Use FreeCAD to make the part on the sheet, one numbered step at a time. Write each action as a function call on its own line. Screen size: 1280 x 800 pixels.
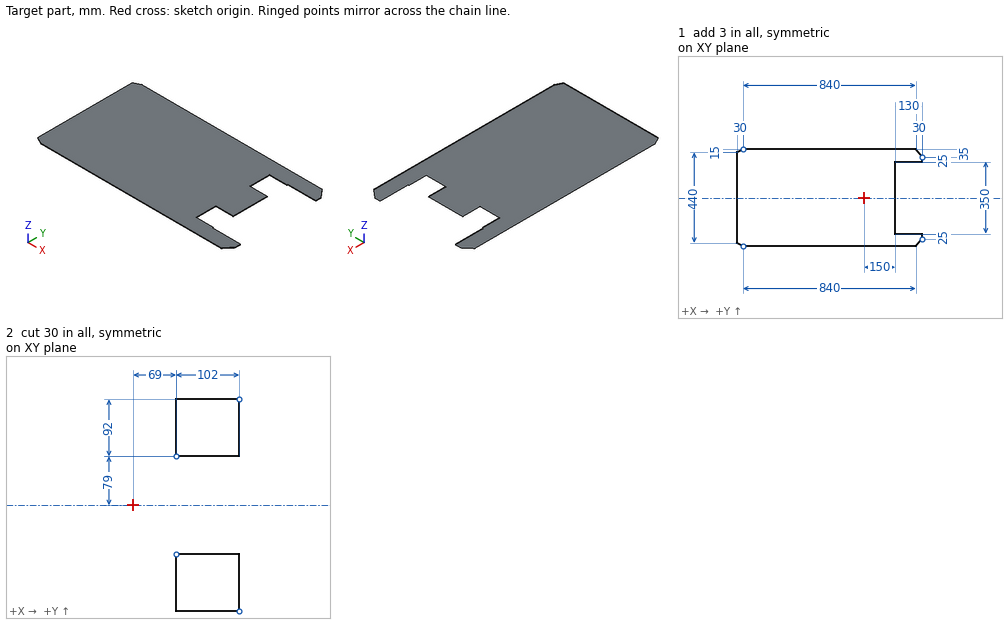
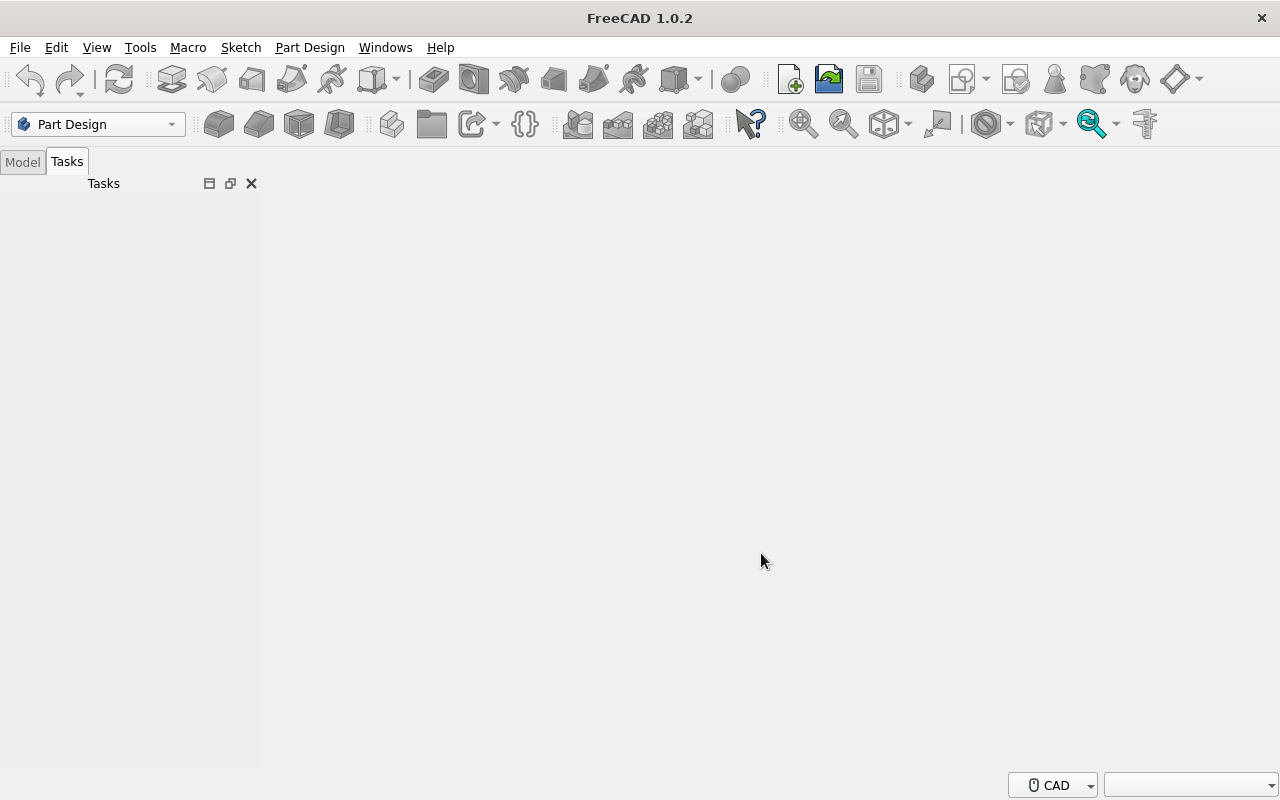
click(790, 80)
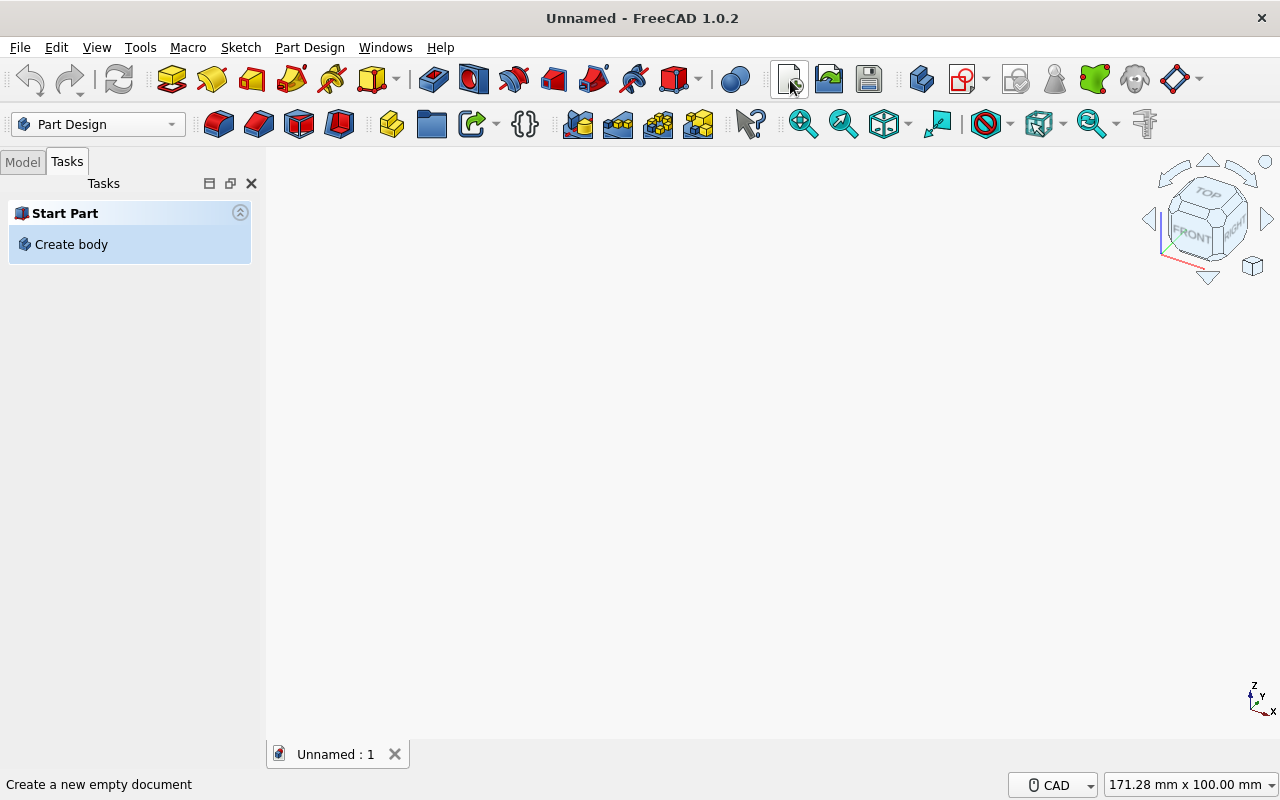
click(962, 80)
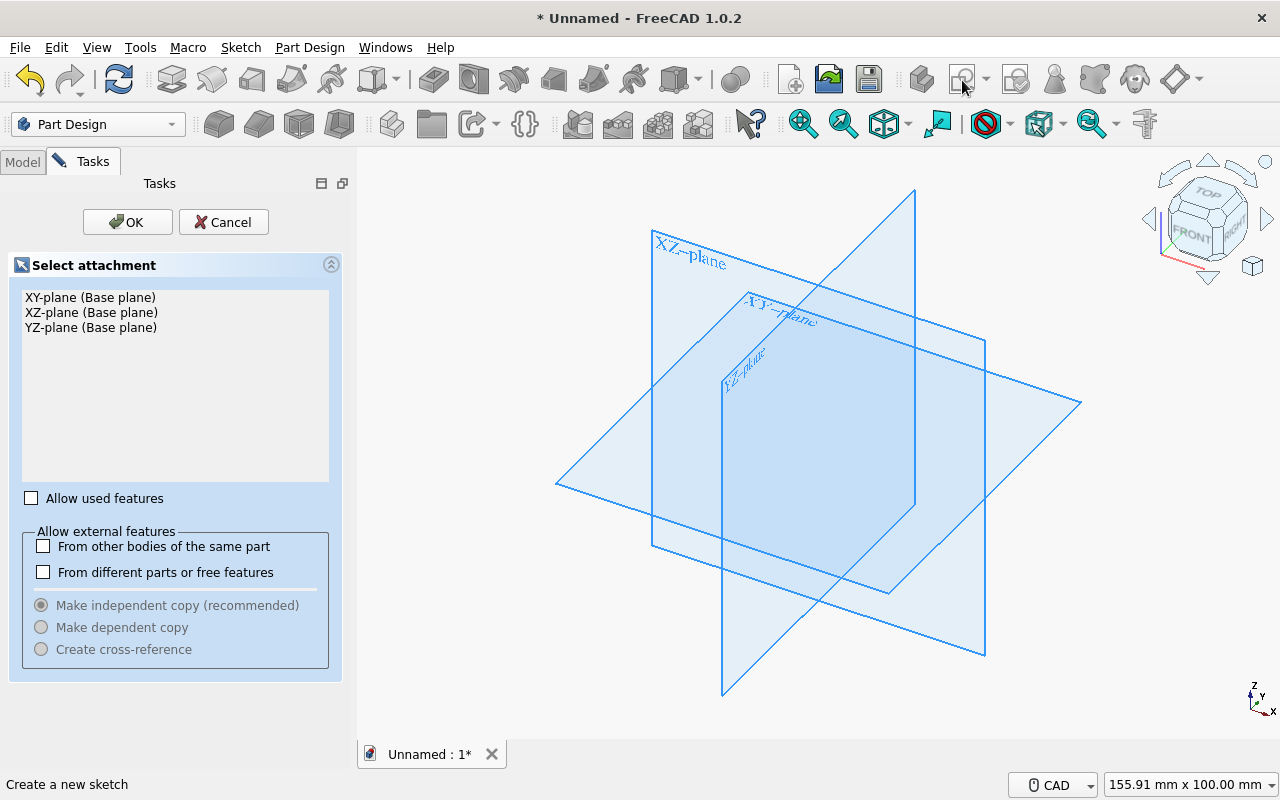
click(82, 298)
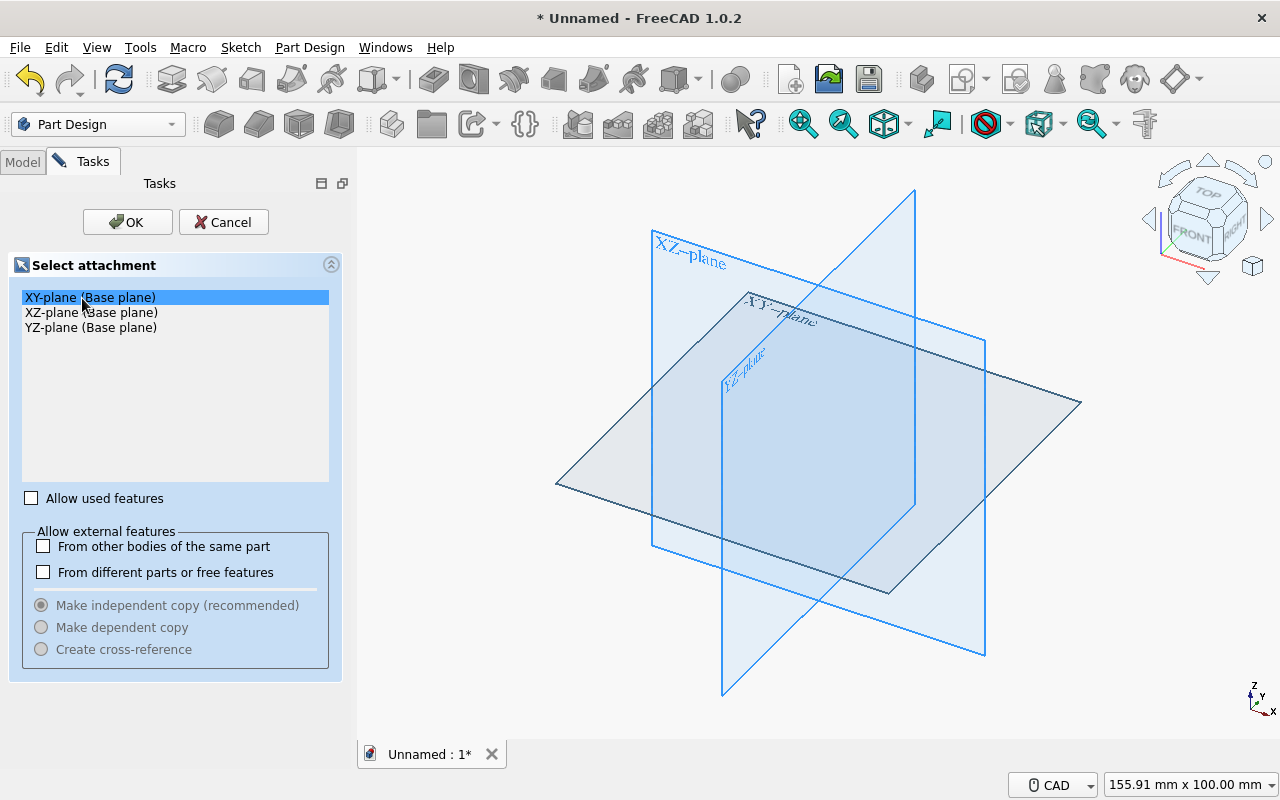
click(128, 222)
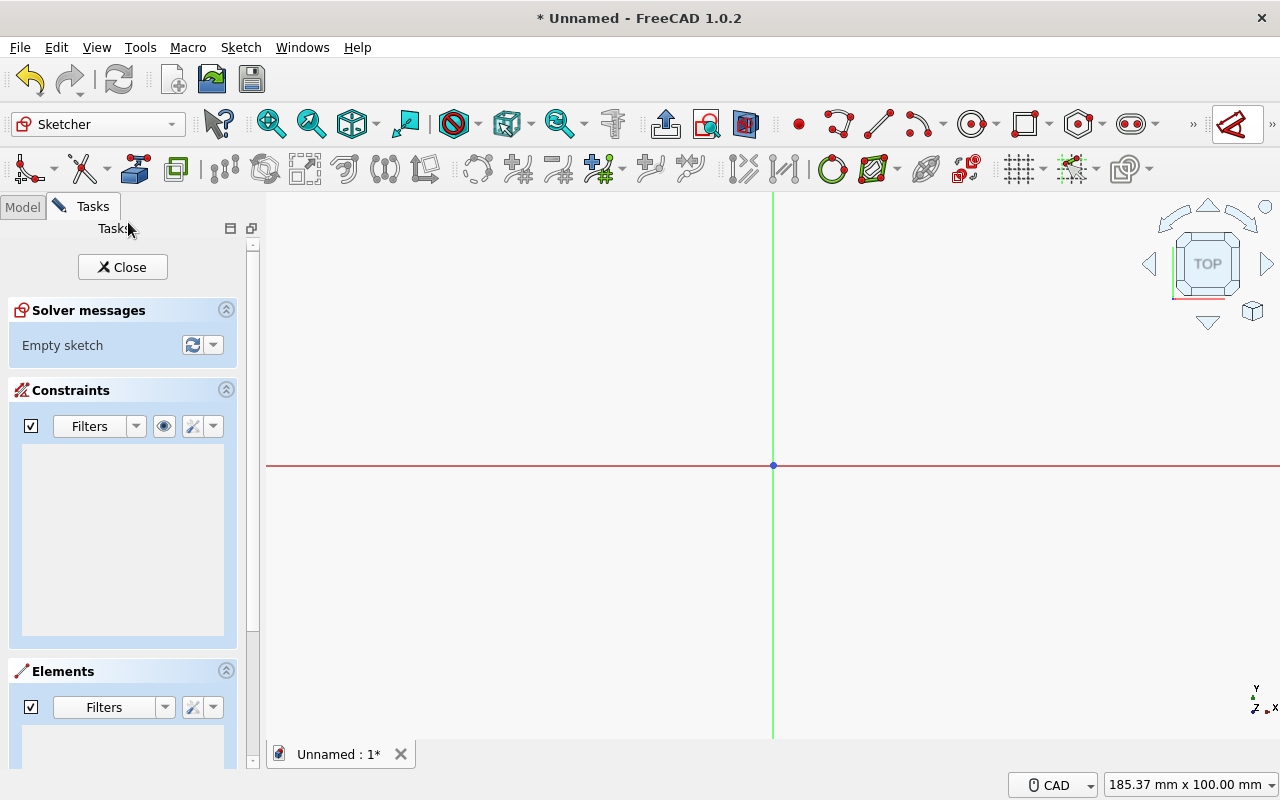
scroll(812, 466, down, 11)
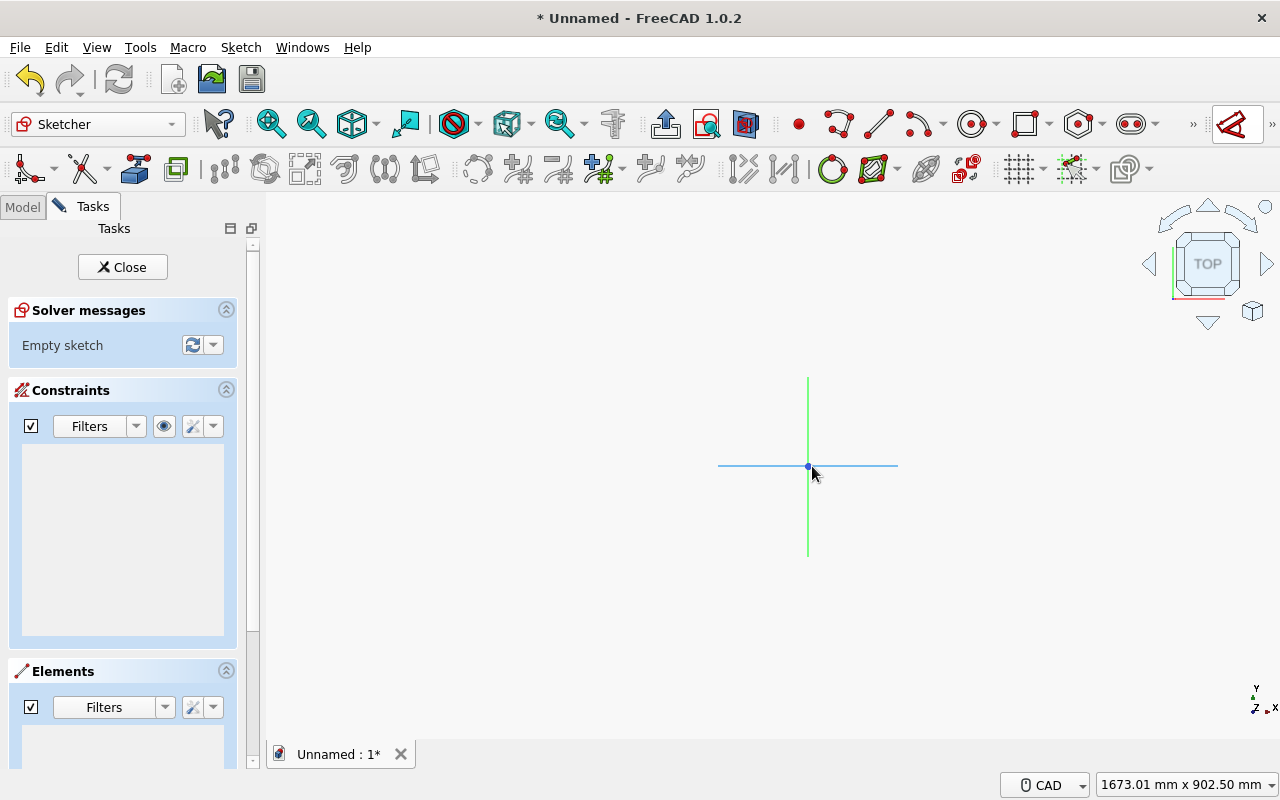
click(840, 124)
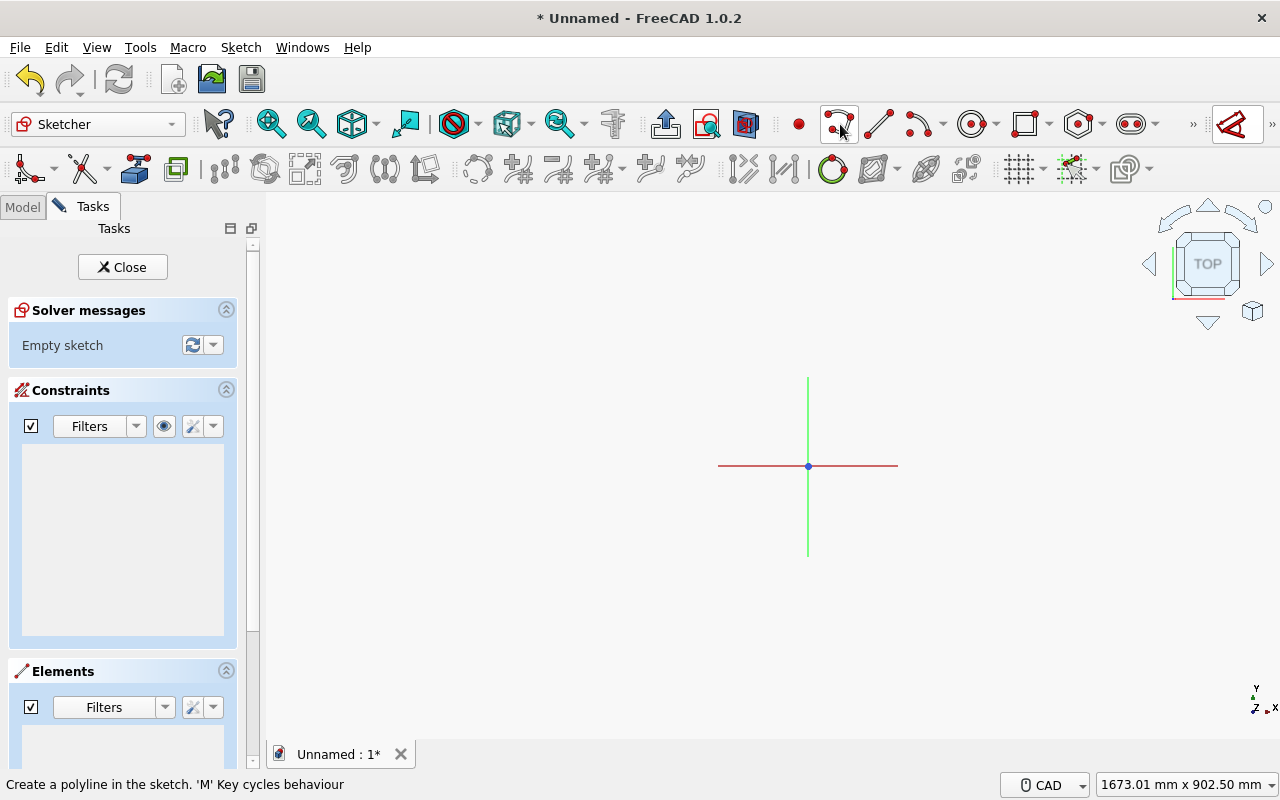
click(899, 572)
click(899, 360)
click(978, 360)
click(978, 345)
click(960, 324)
click(451, 324)
click(432, 333)
click(432, 600)
click(451, 609)
click(960, 609)
click(978, 588)
click(978, 572)
click(899, 573)
key(Escape)
key(Escape)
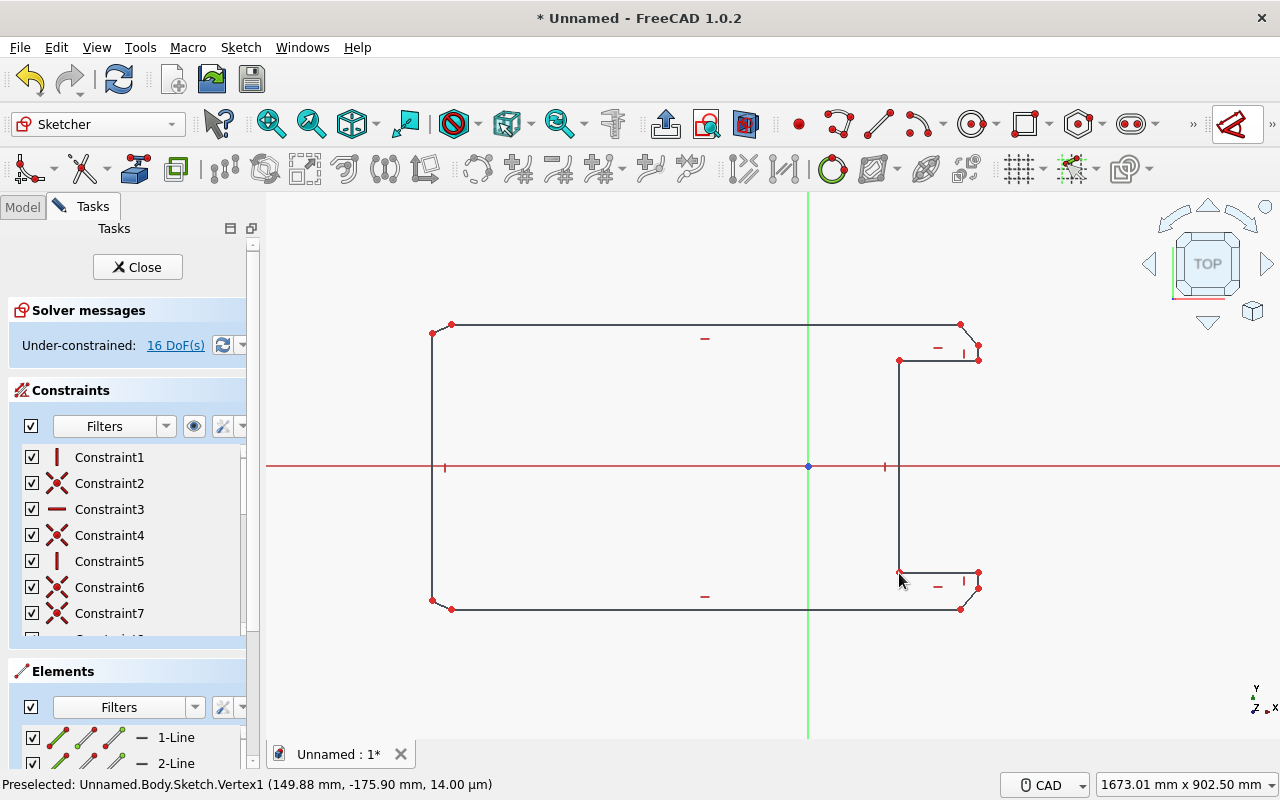
click(451, 325)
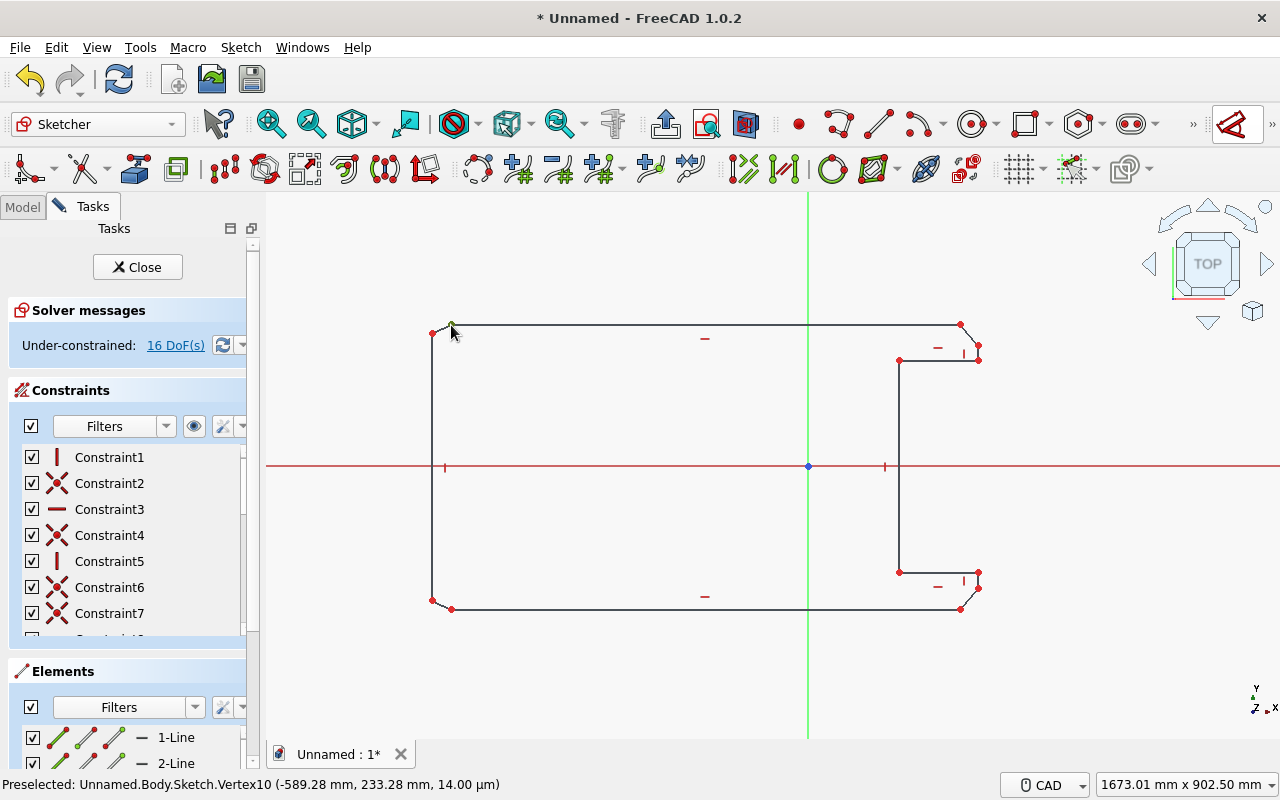
click(451, 610)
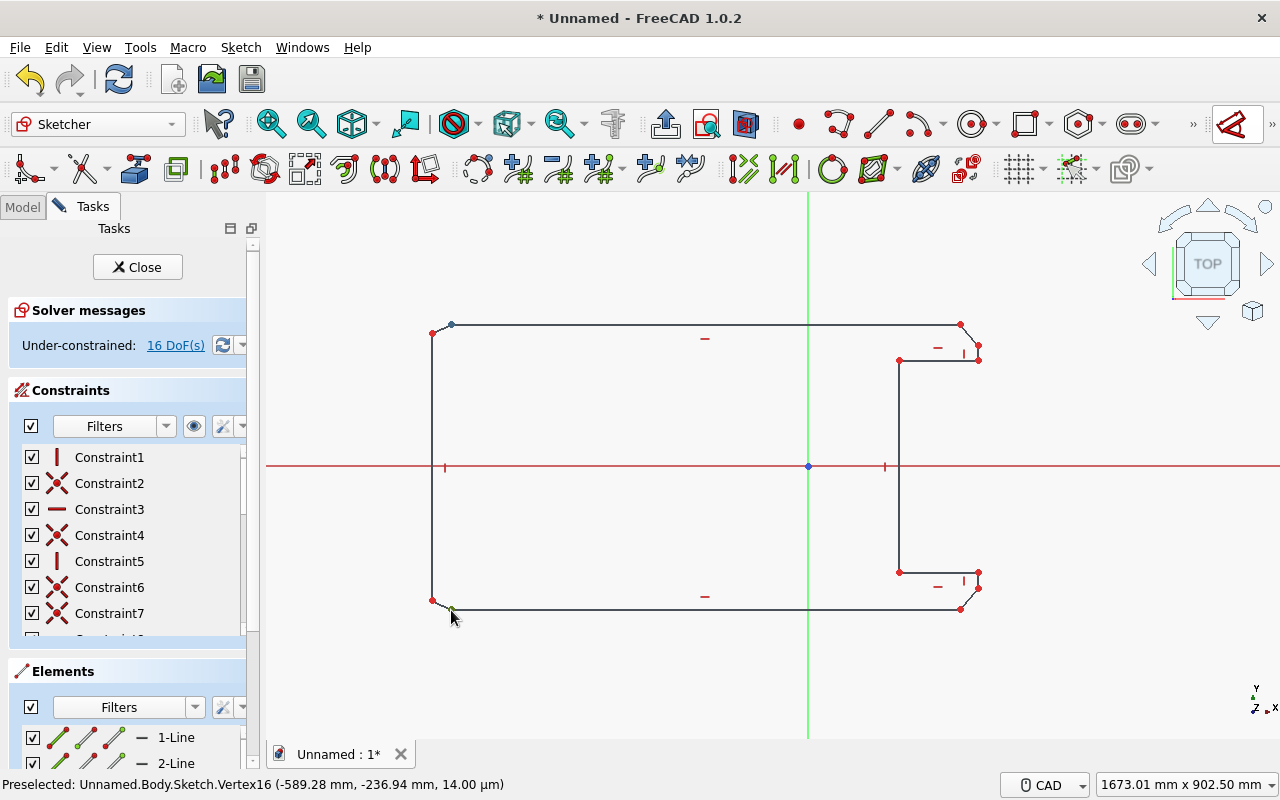
click(353, 466)